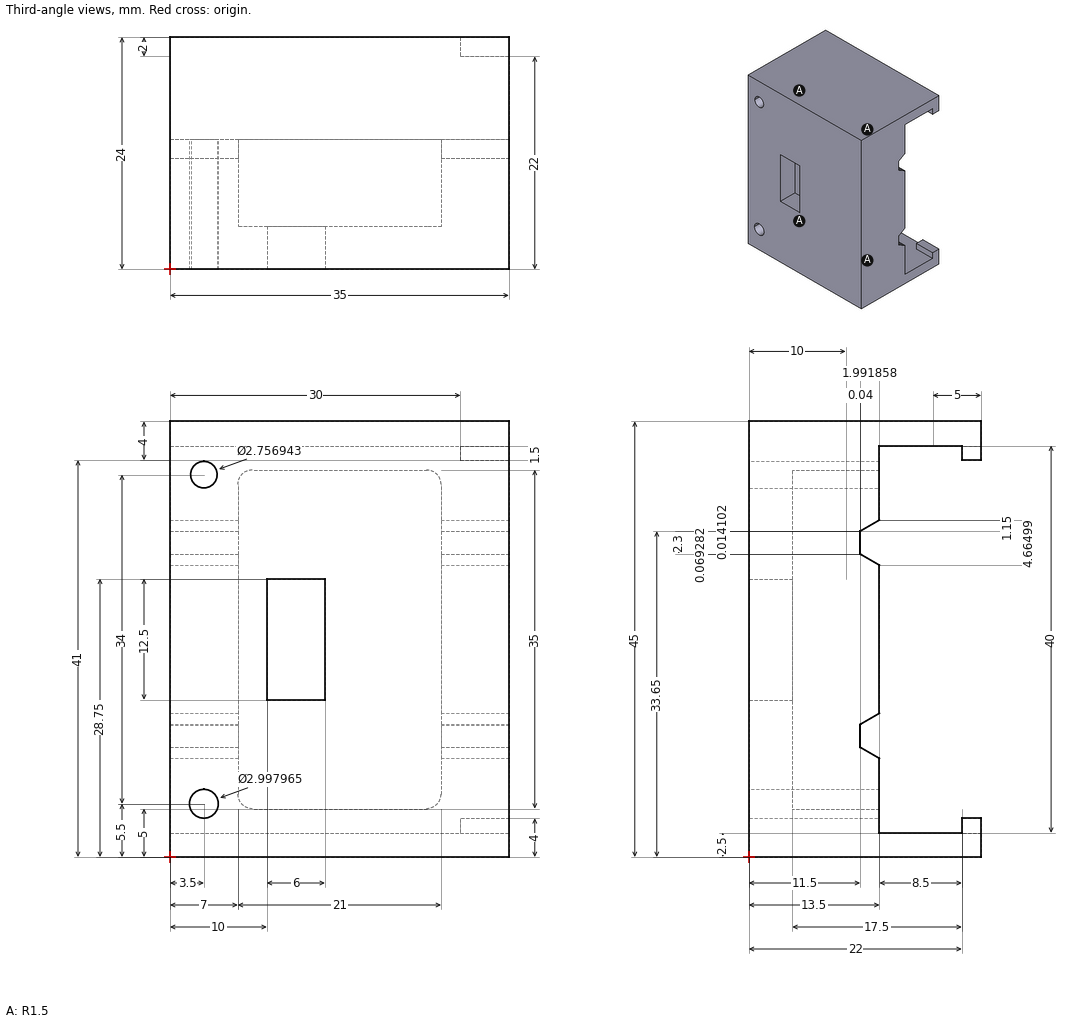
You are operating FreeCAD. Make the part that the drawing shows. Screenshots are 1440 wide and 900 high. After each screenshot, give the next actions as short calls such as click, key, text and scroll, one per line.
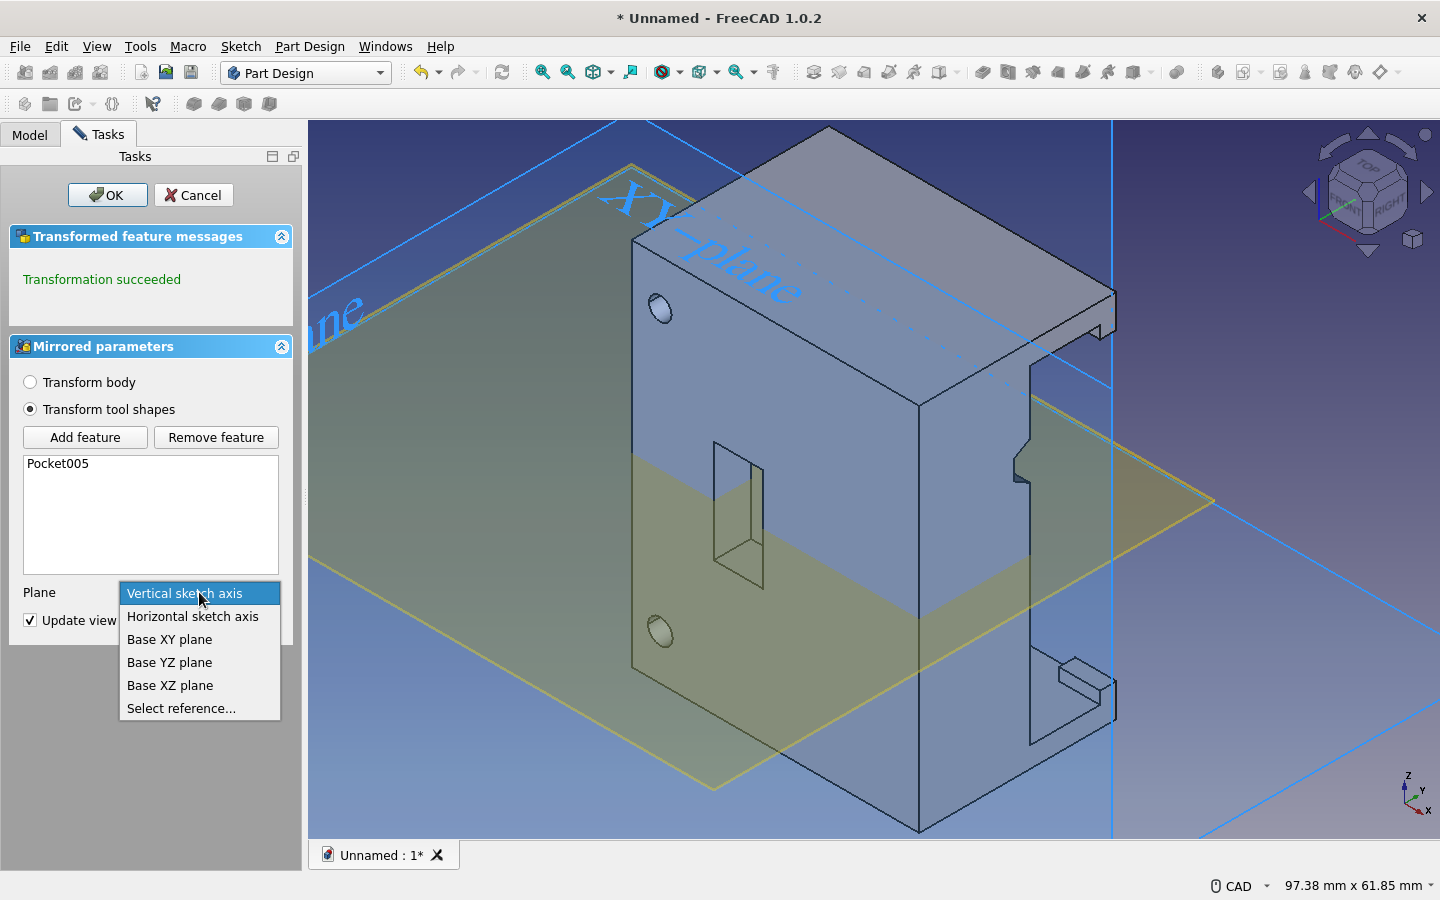
click(198, 708)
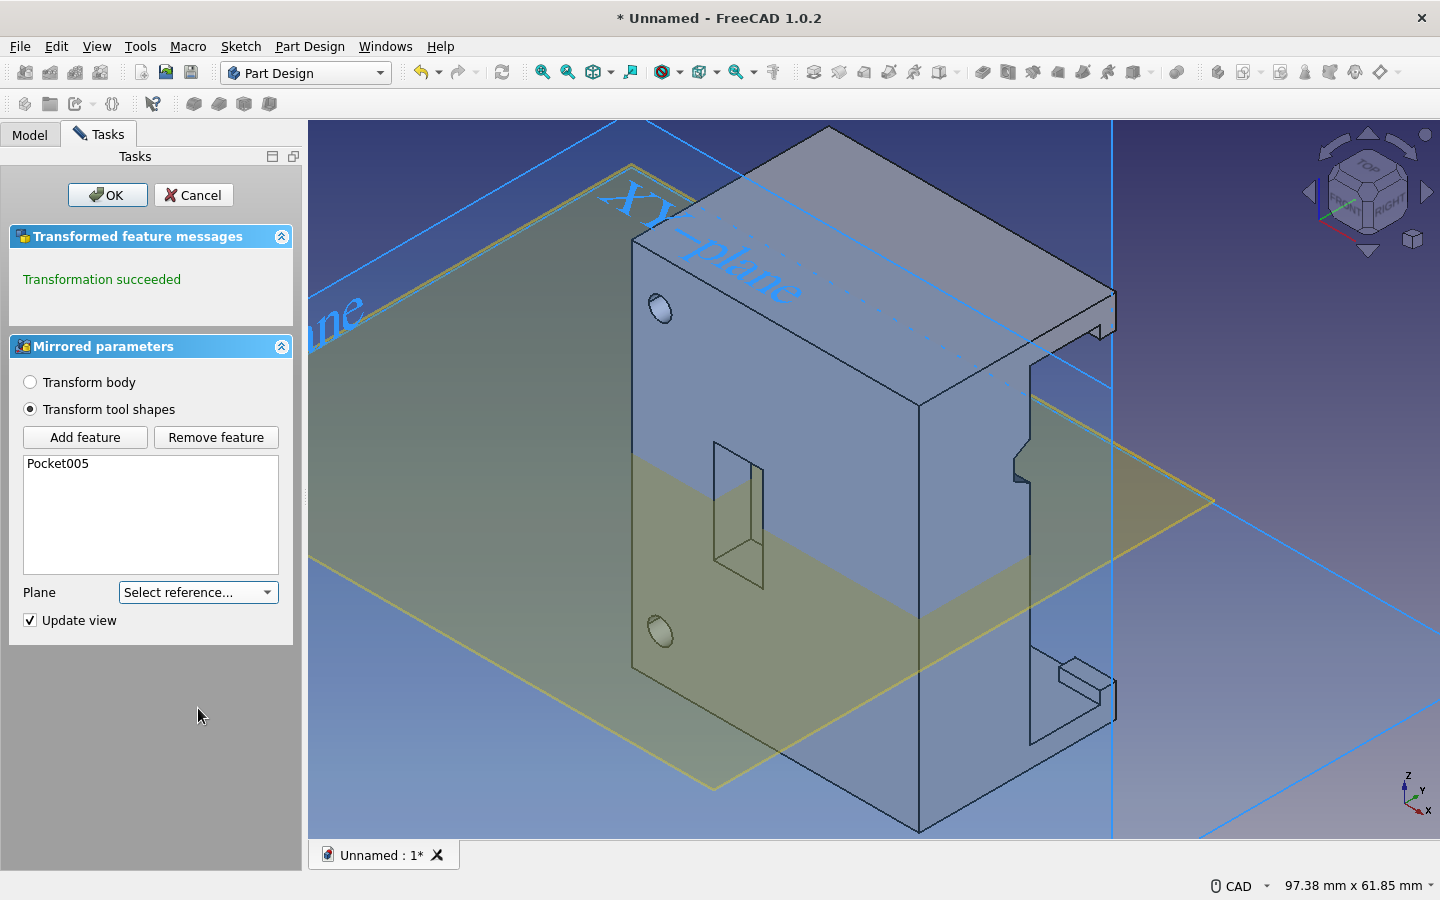
click(30, 134)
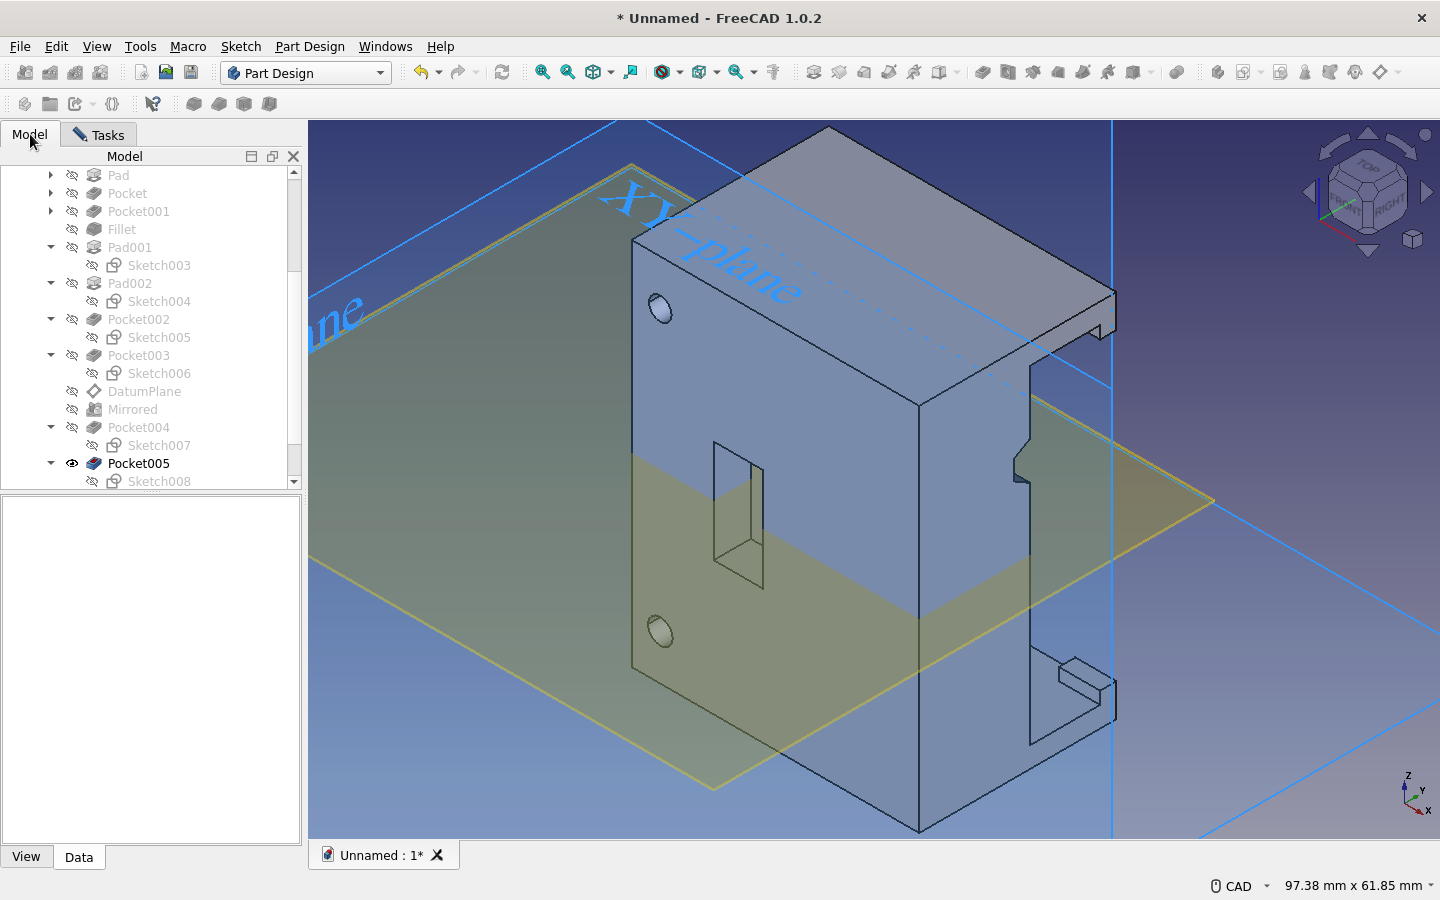
scroll(141, 333, down, 3)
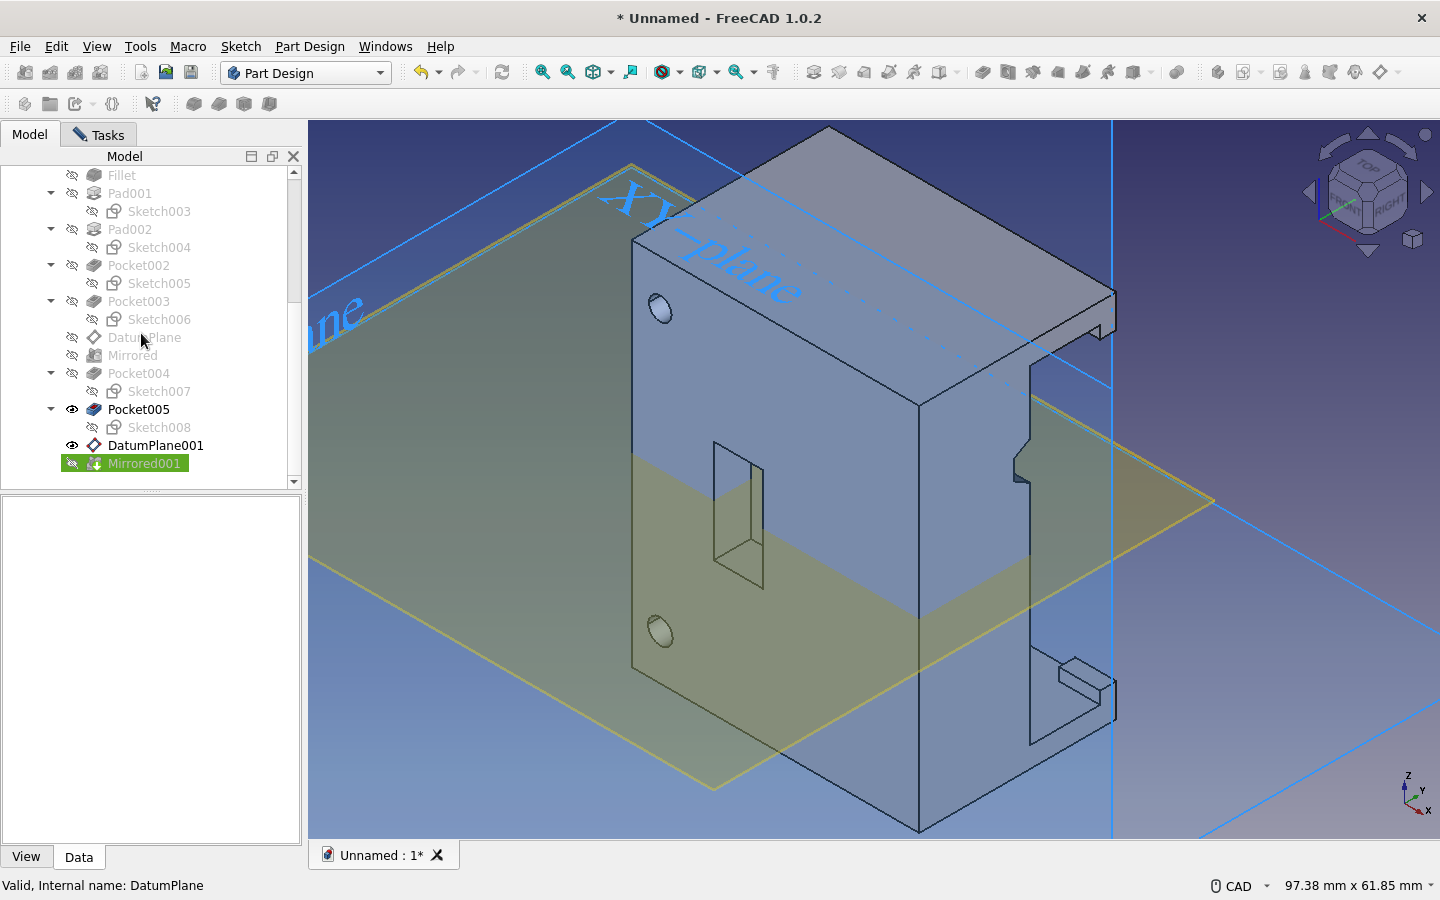
click(117, 445)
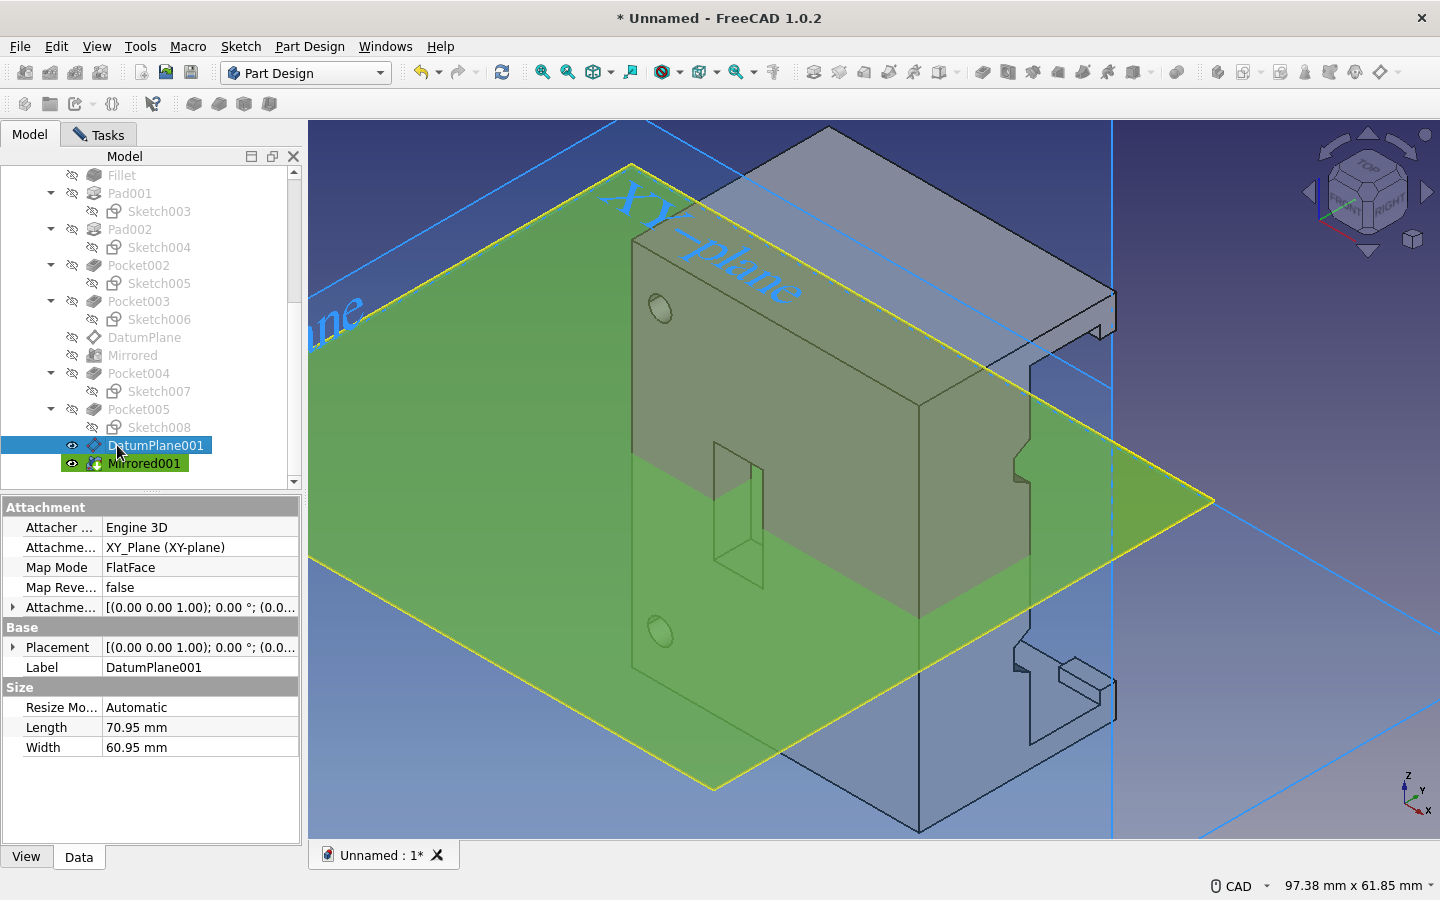
click(98, 134)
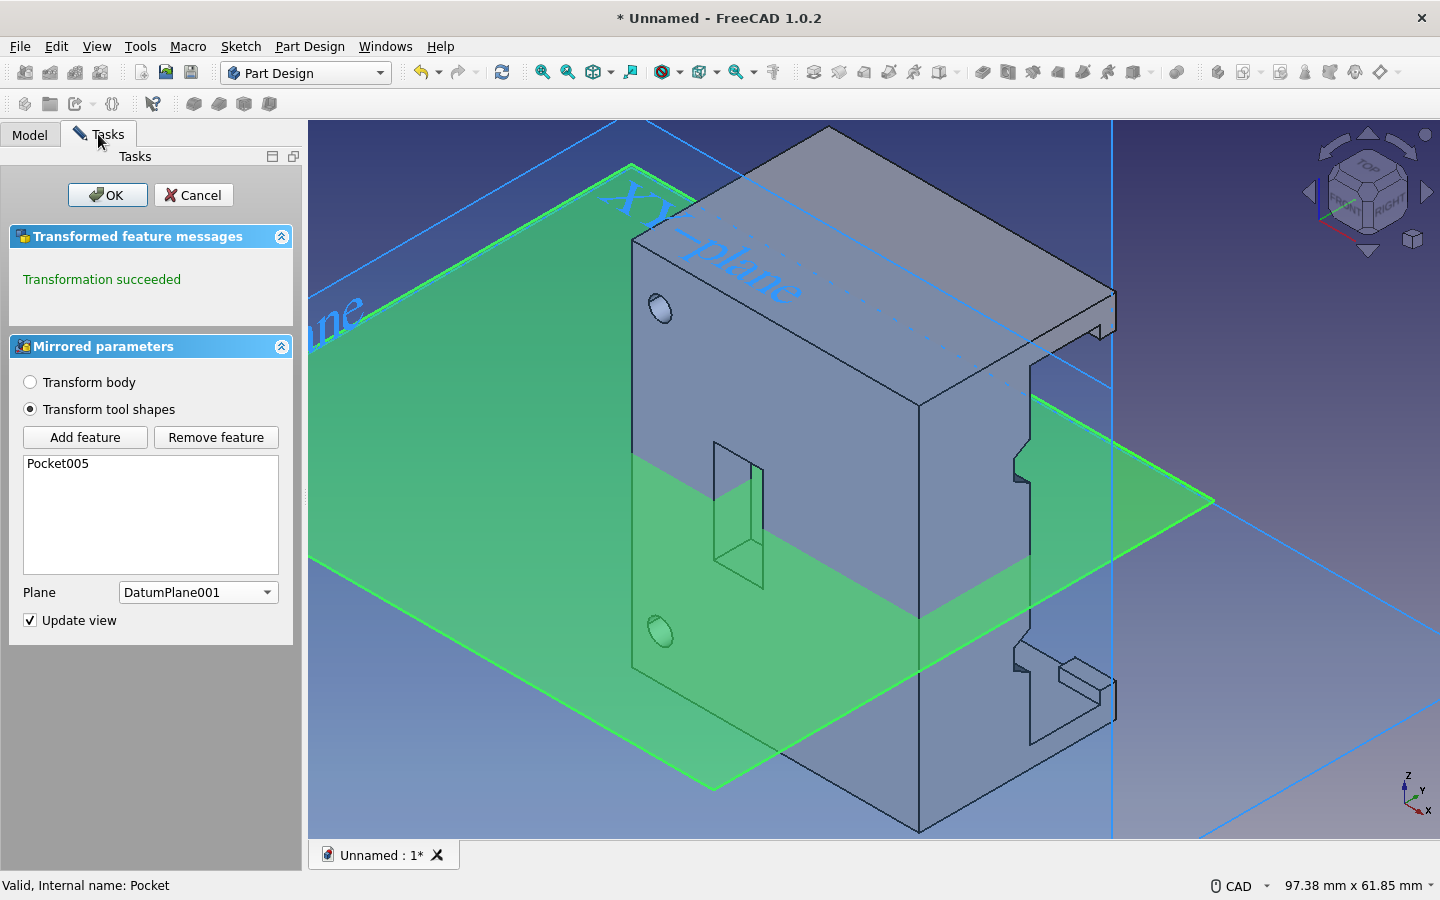
click(108, 195)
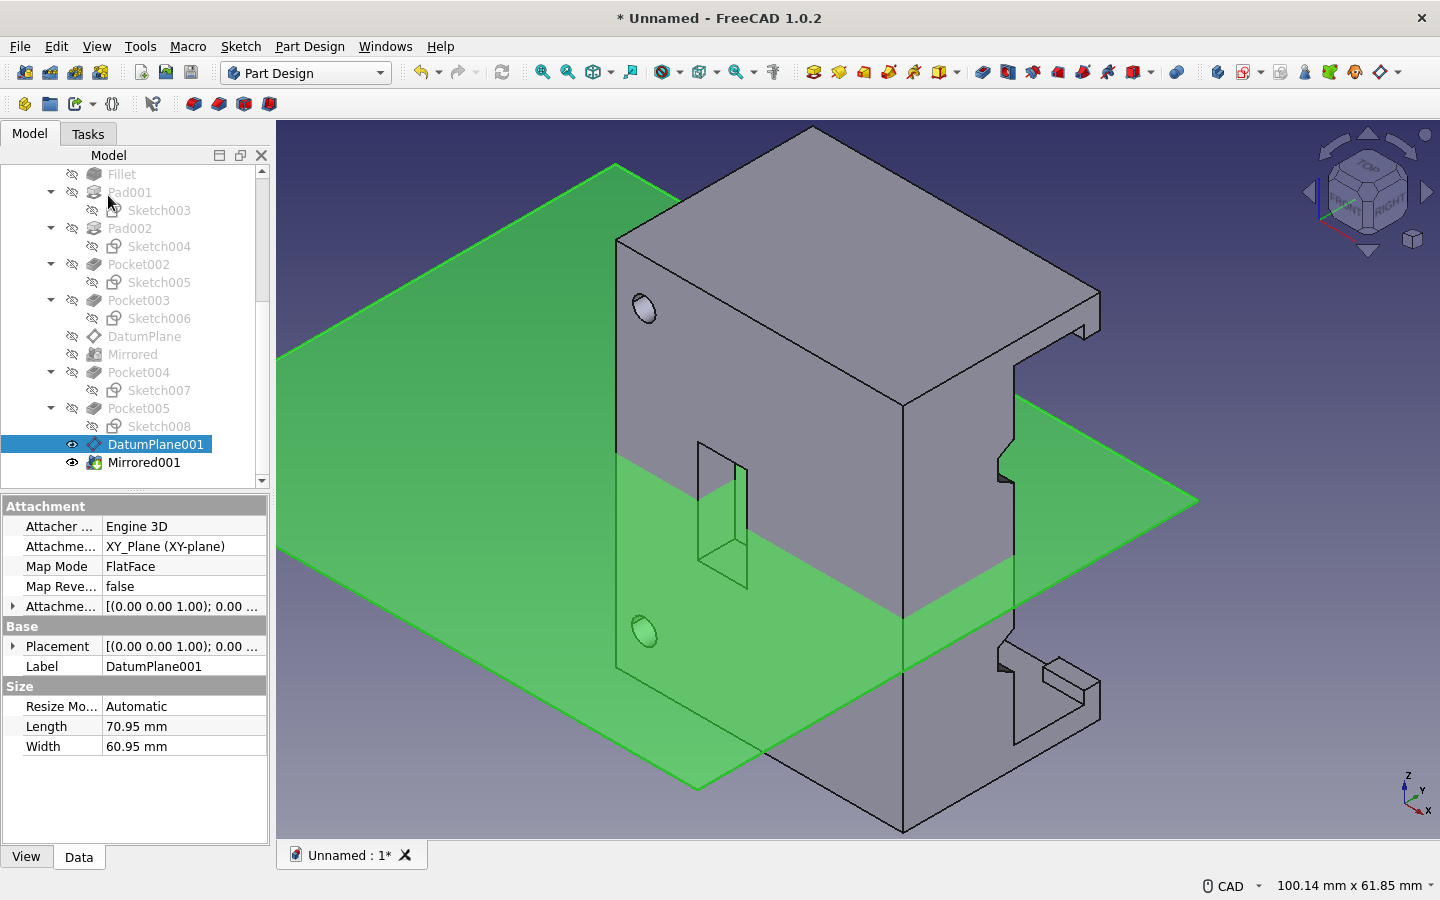
click(117, 444)
key(space)